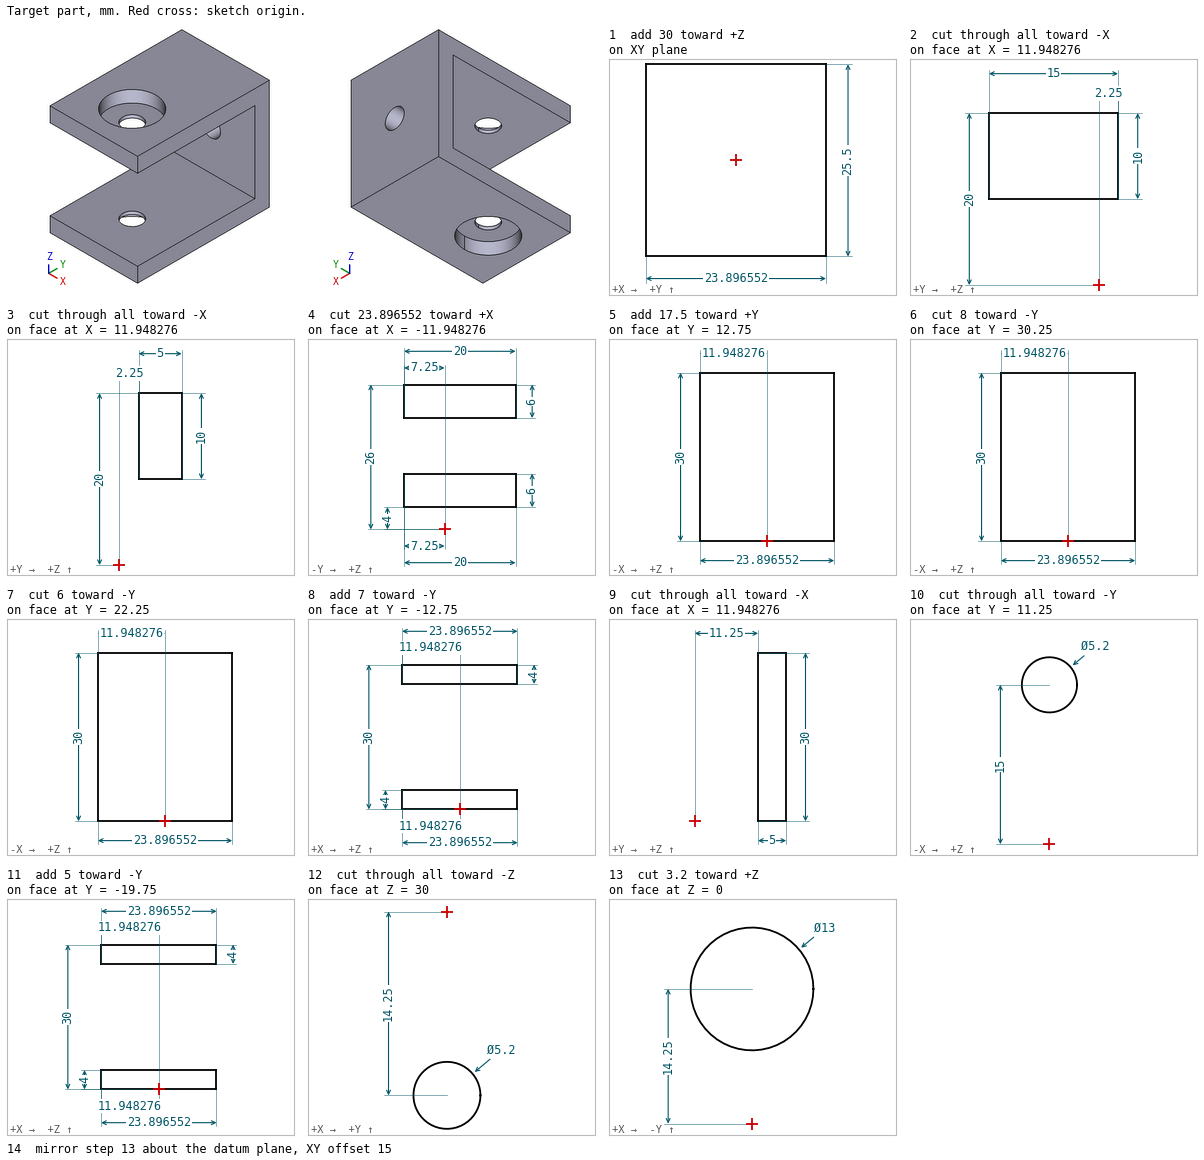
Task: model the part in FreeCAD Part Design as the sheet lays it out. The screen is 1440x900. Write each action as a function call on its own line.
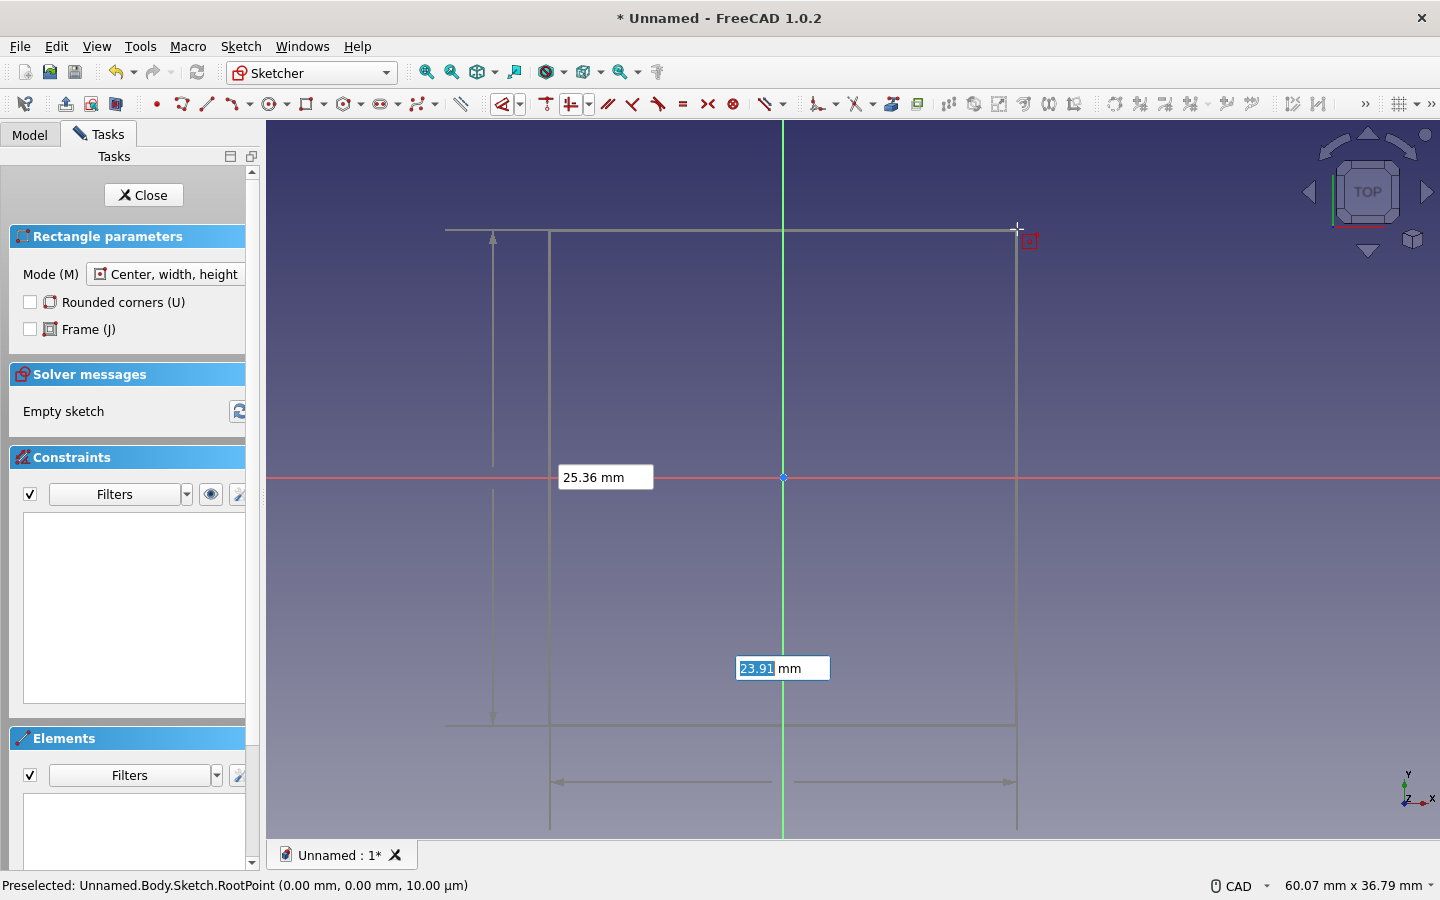
text(23.896552)
key(Tab)
text(25.5)
key(Return)
key(Escape)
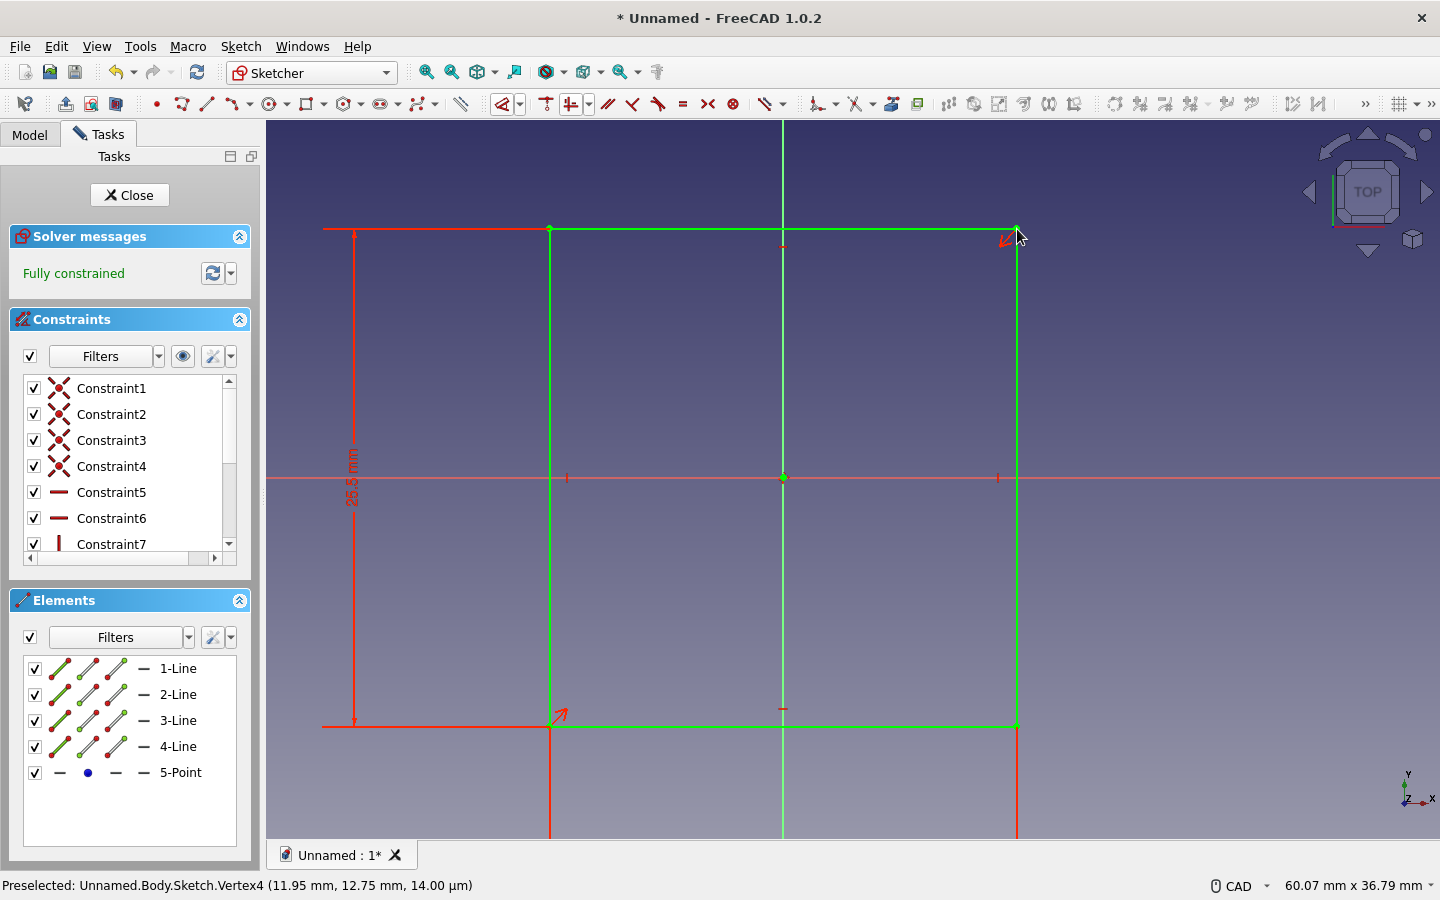
click(130, 195)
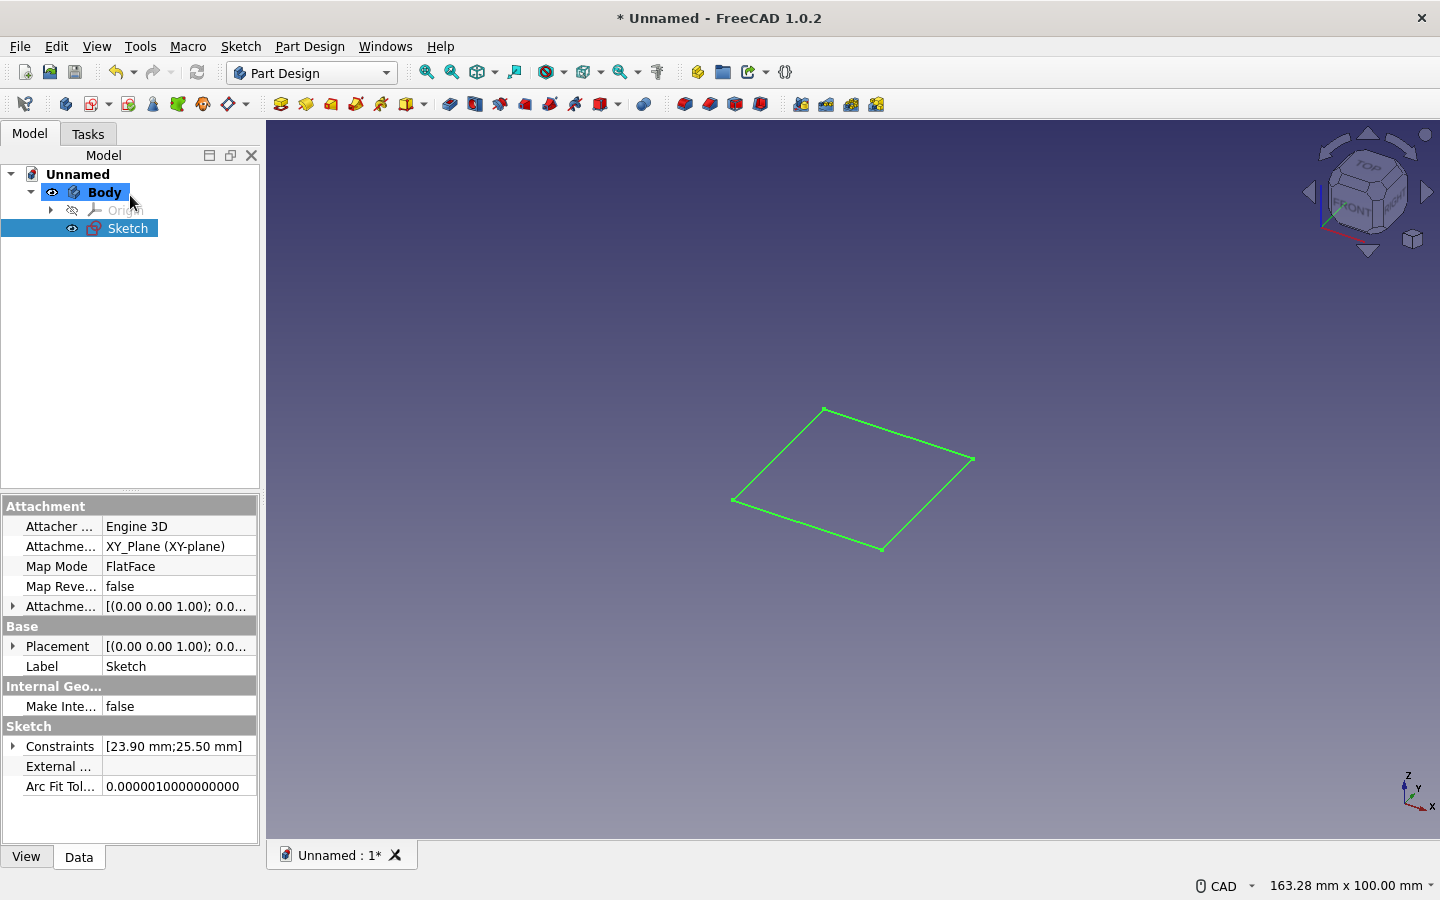
click(281, 104)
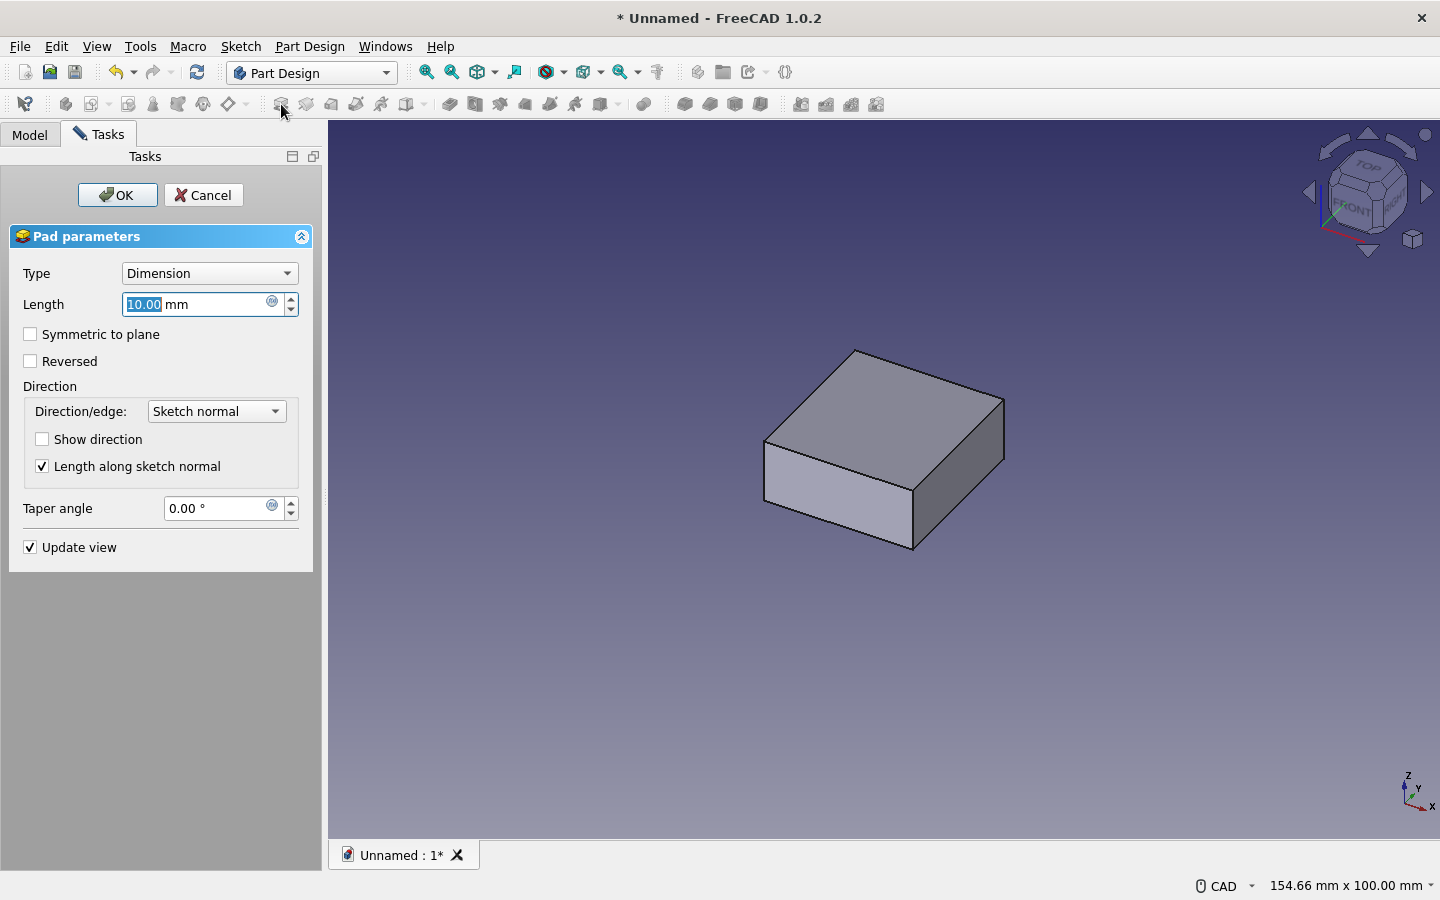
text(30)
key(Tab)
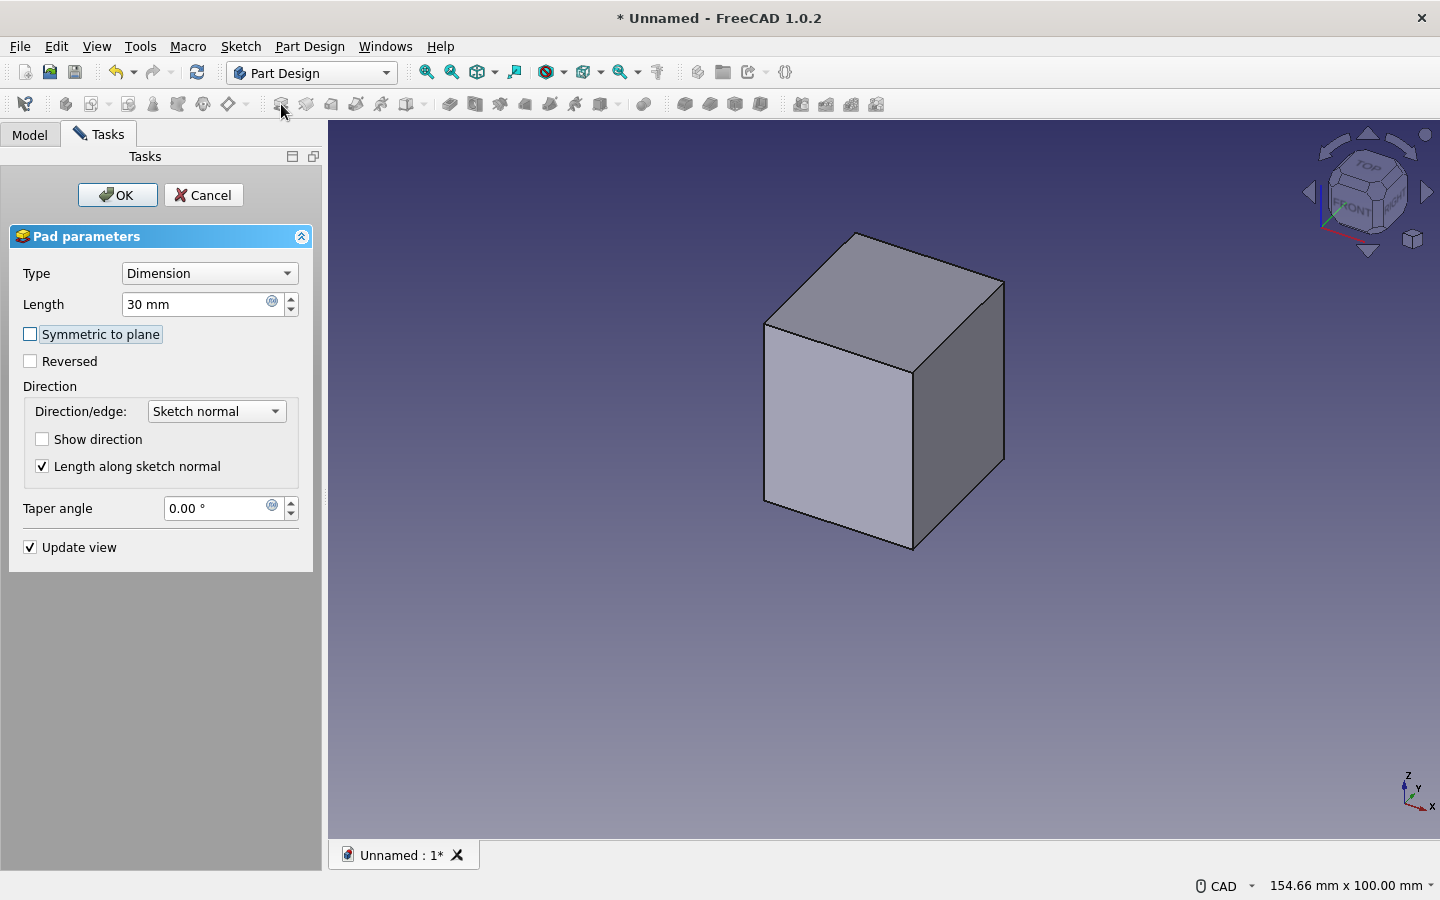
click(118, 195)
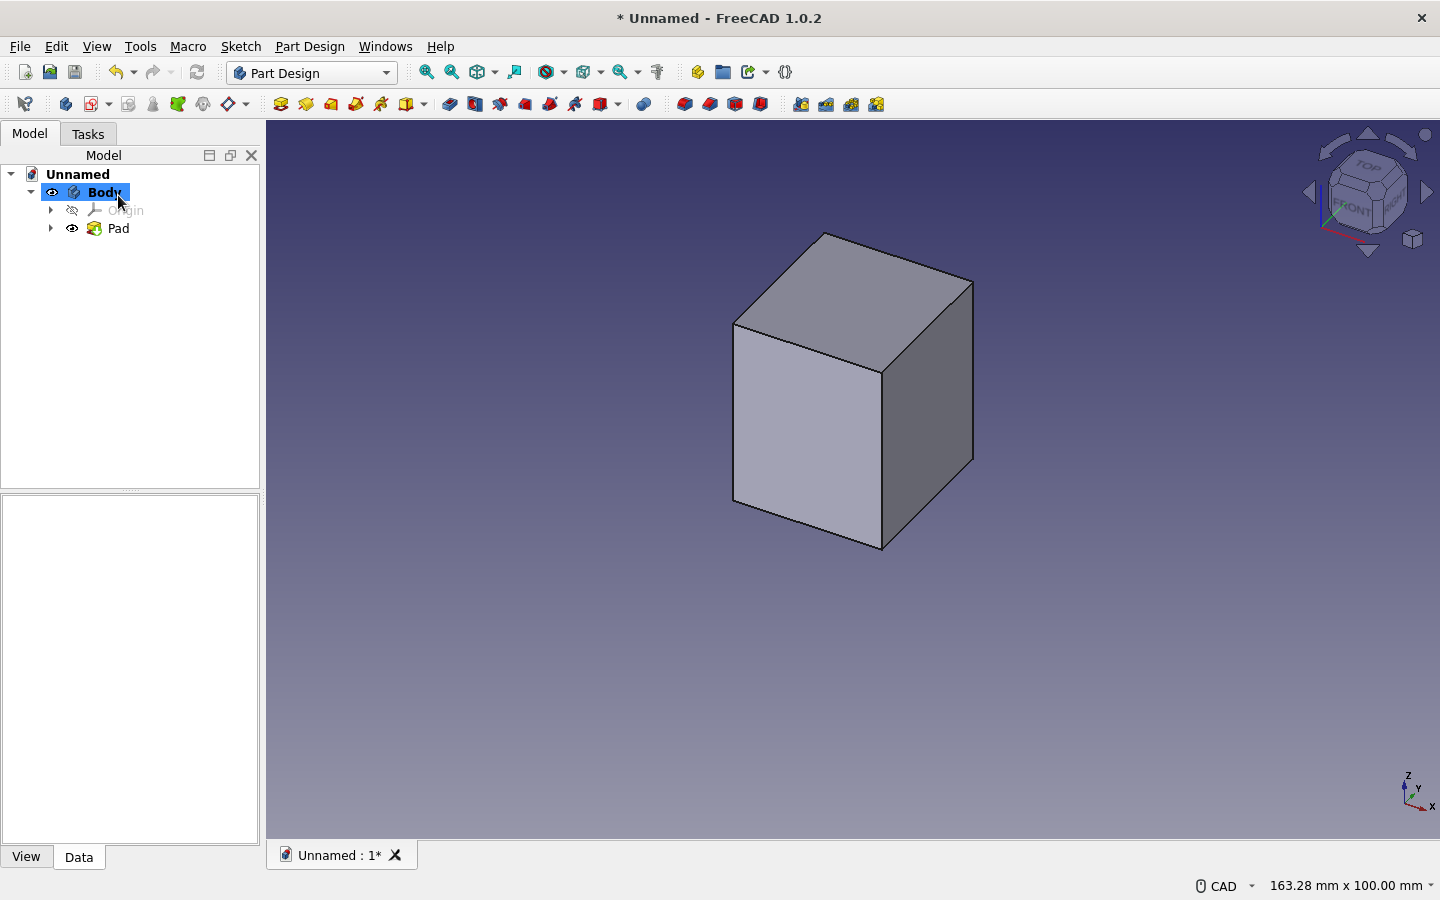
key(v)
key(f)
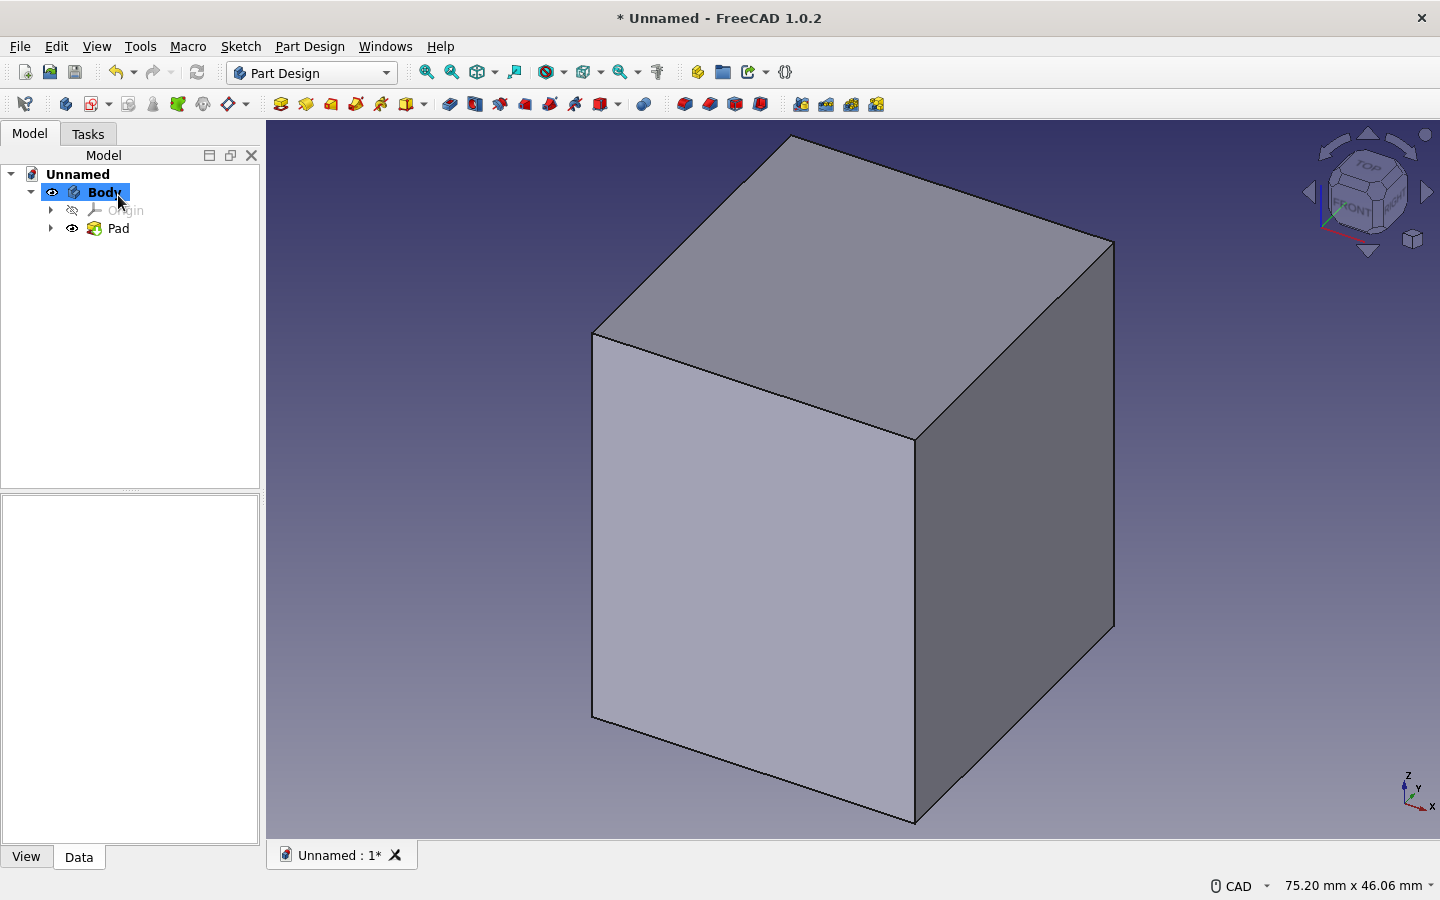
click(1015, 532)